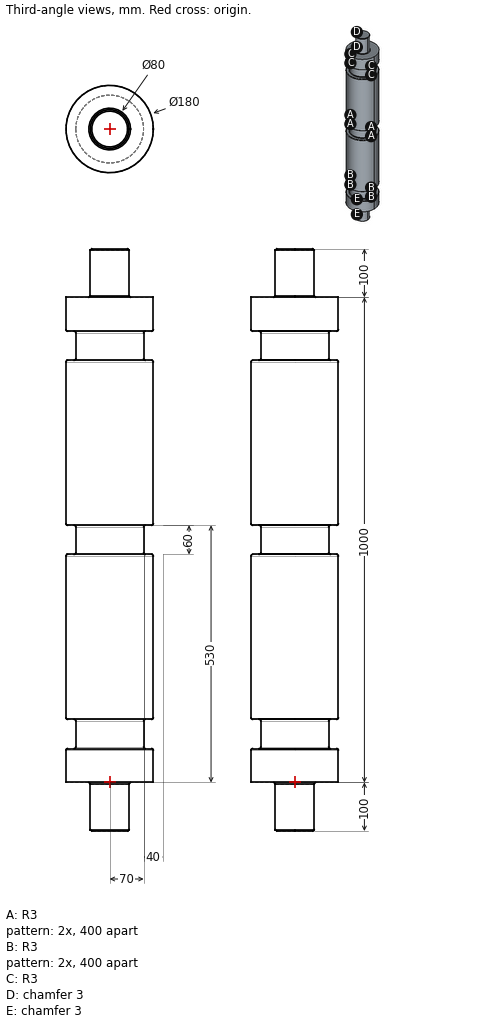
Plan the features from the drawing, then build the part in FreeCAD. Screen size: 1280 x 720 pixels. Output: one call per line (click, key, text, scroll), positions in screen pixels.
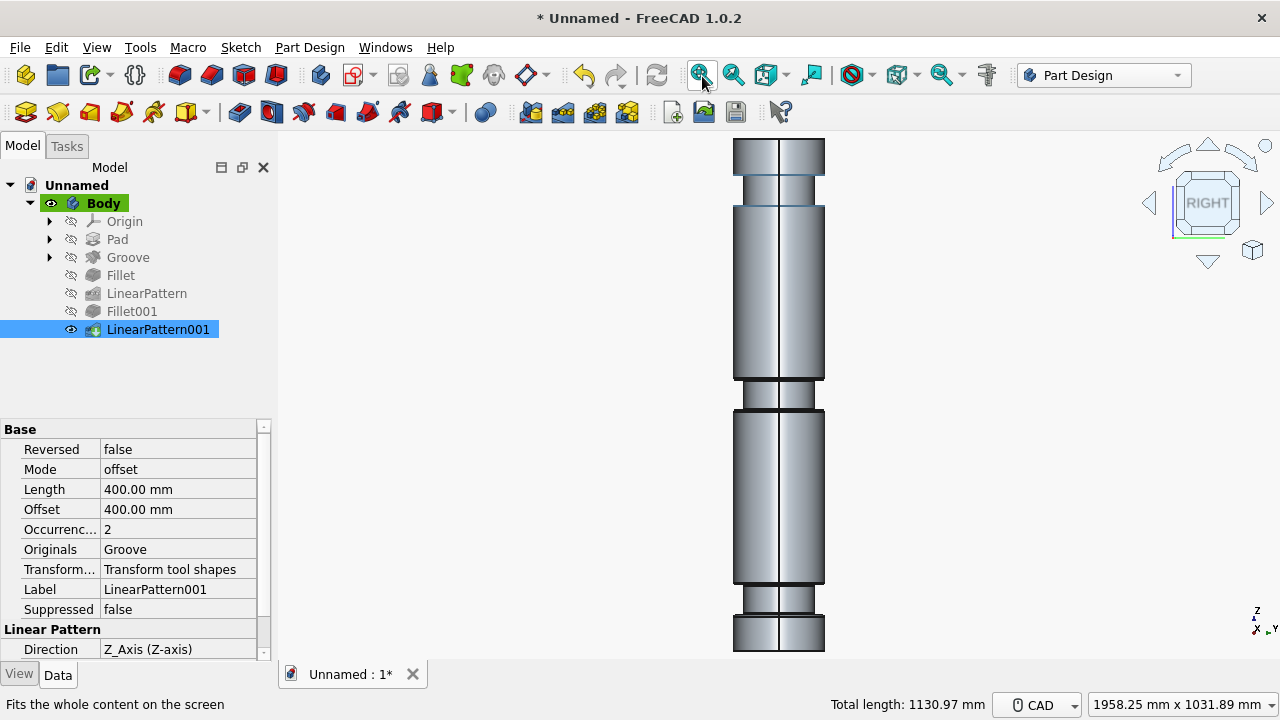
key(5)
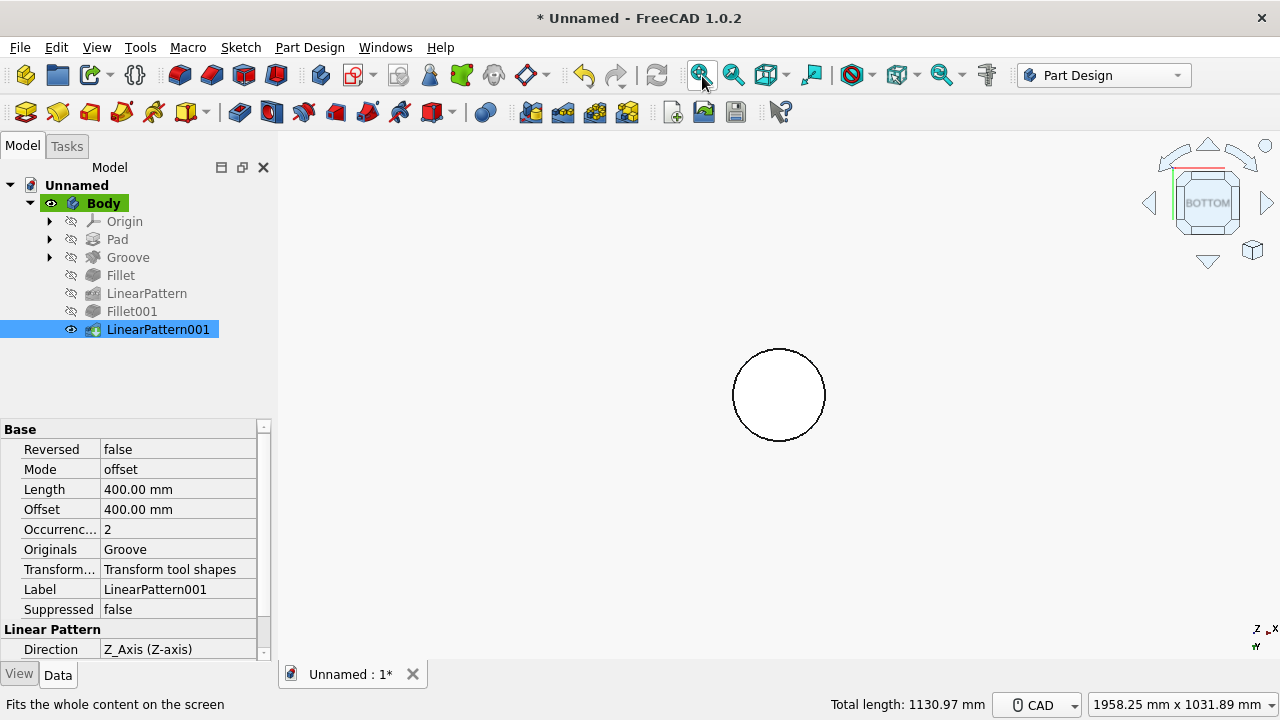
click(702, 76)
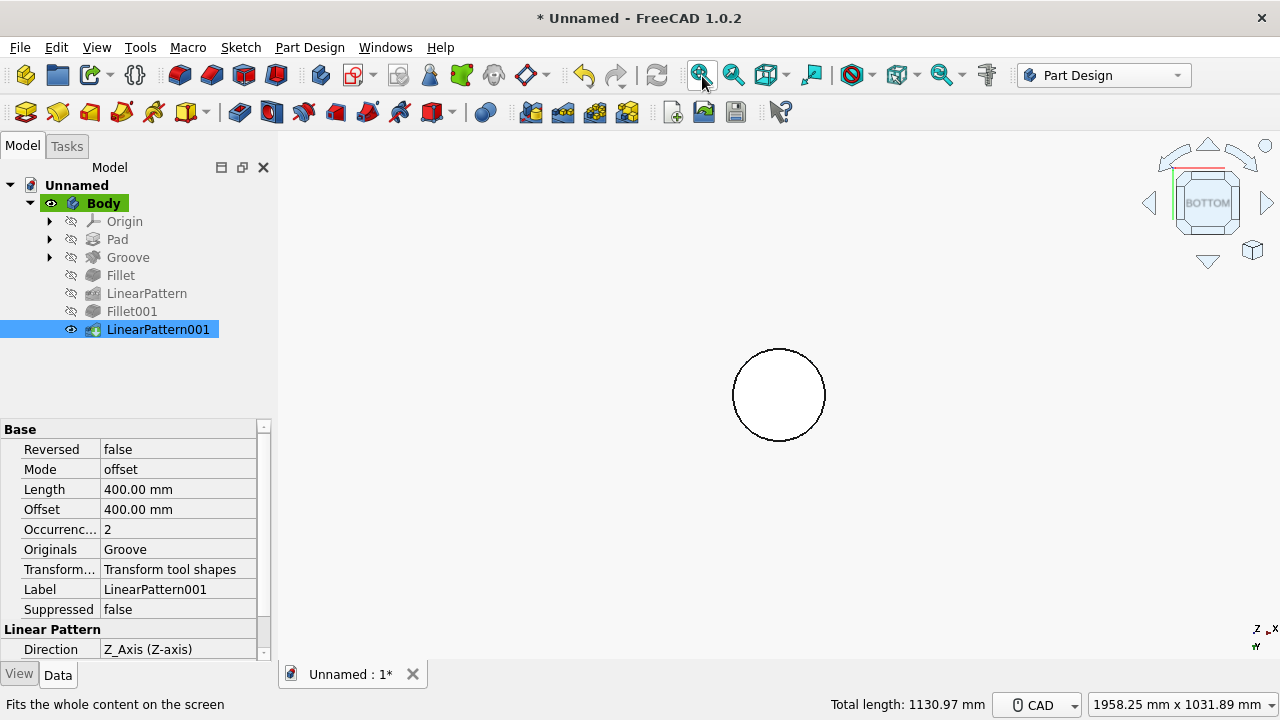
key(4)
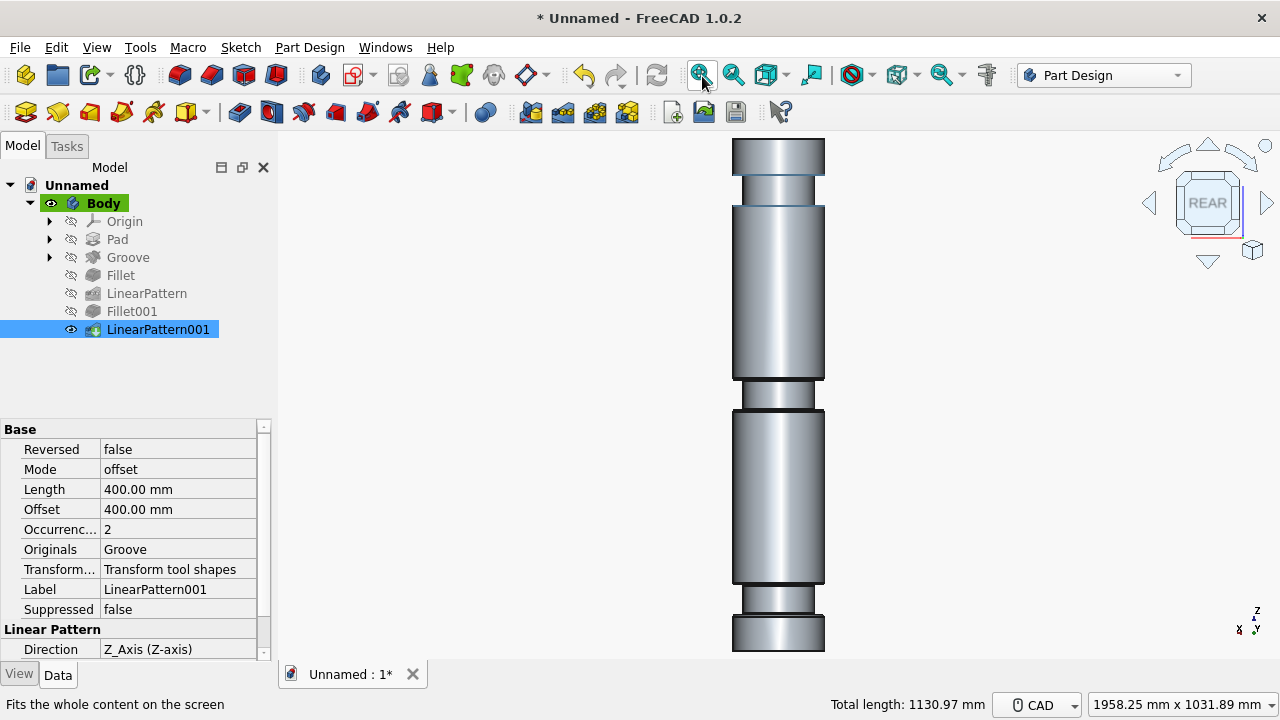
key(6)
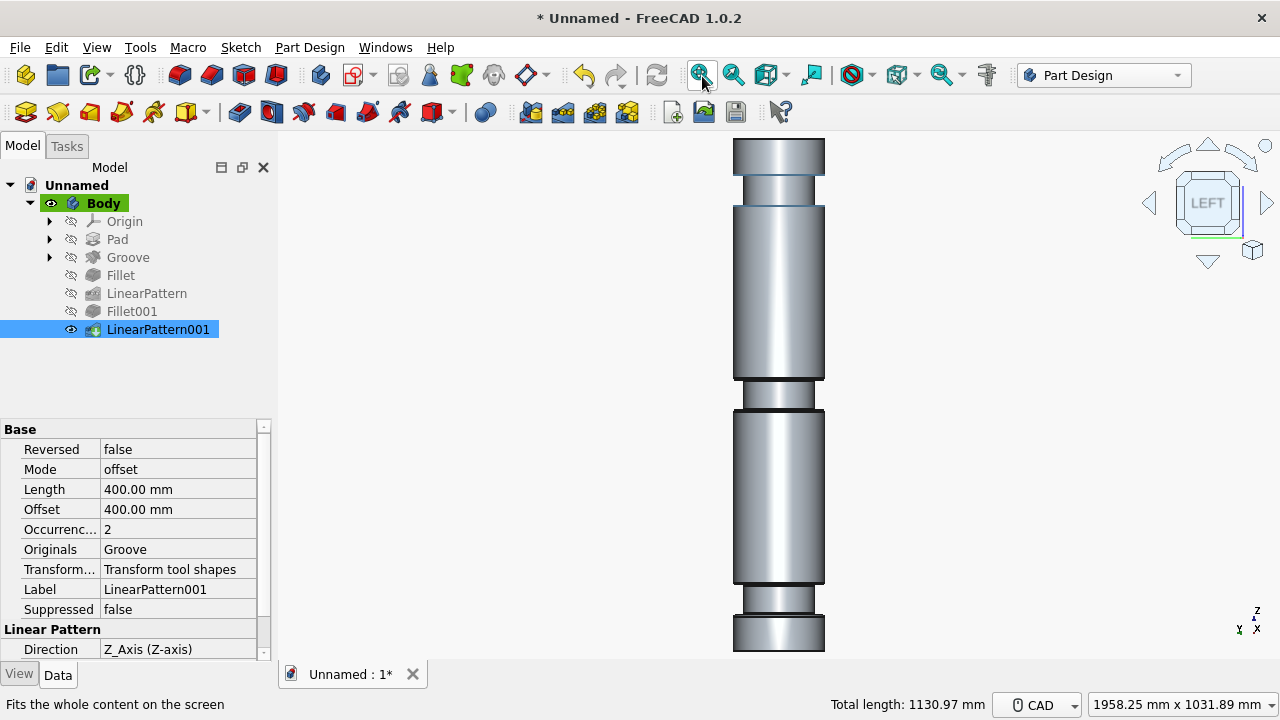
key(v)
key(3)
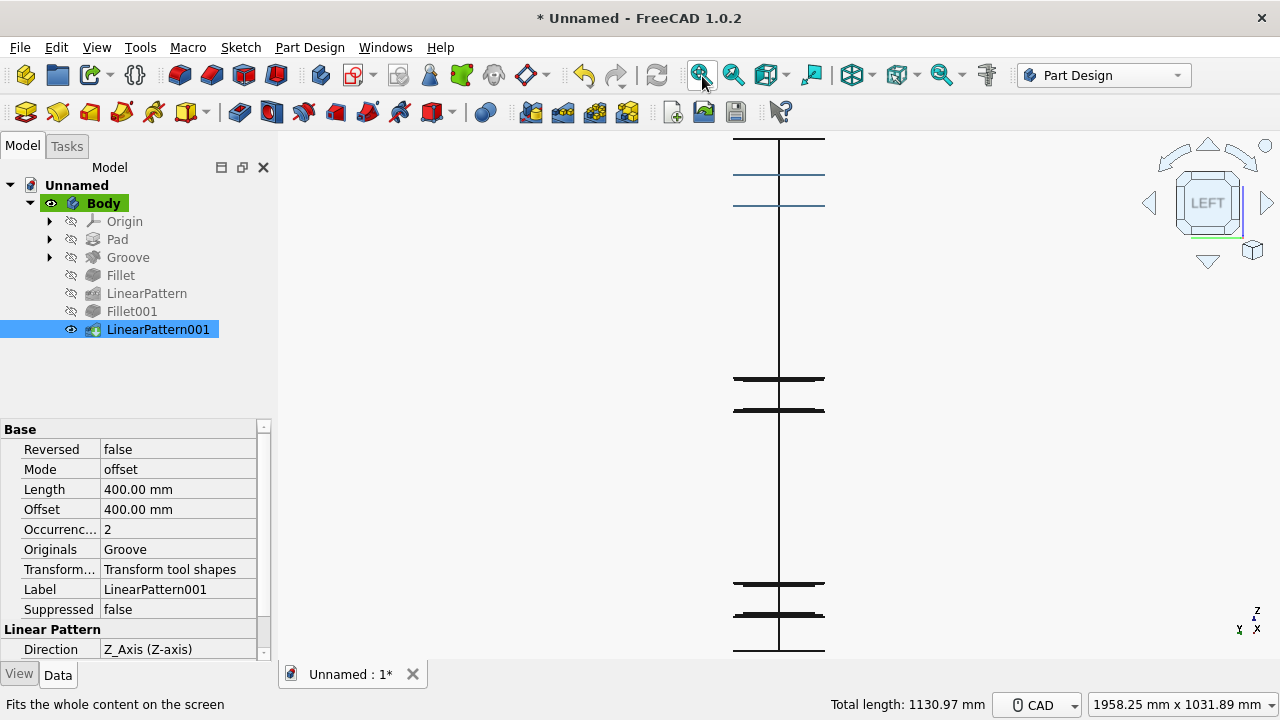
key(0)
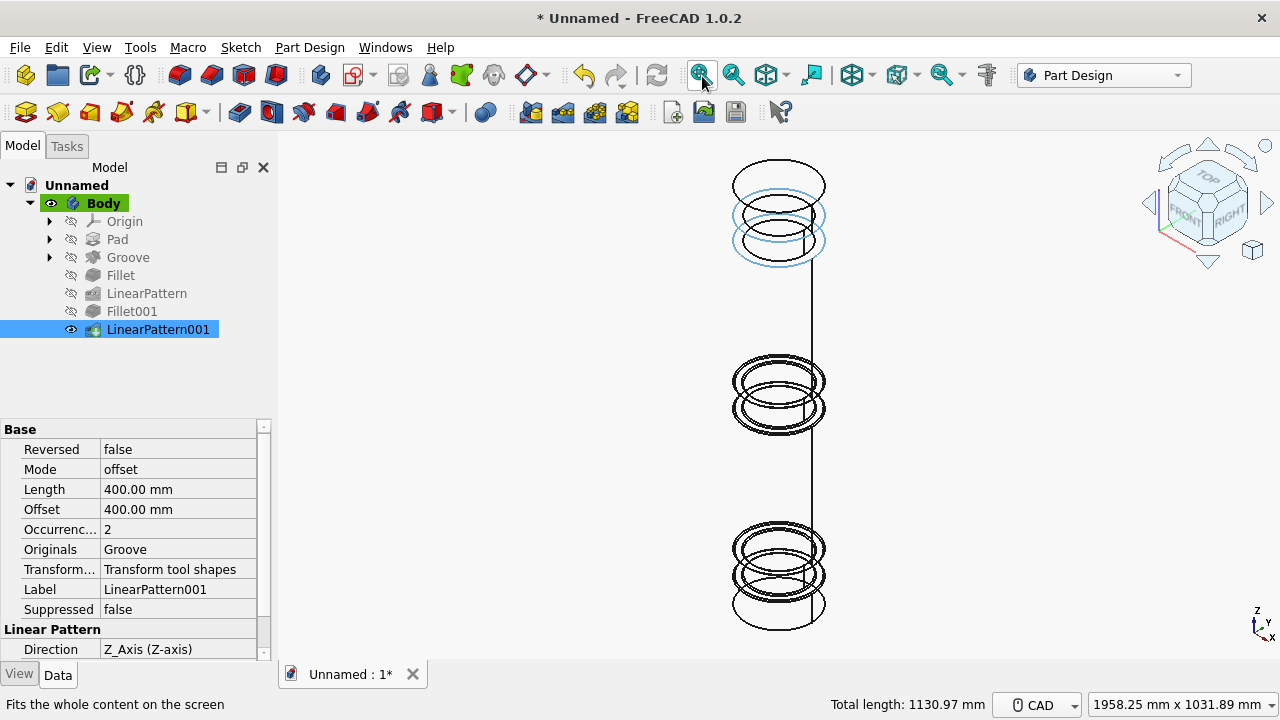
click(754, 200, ctrl)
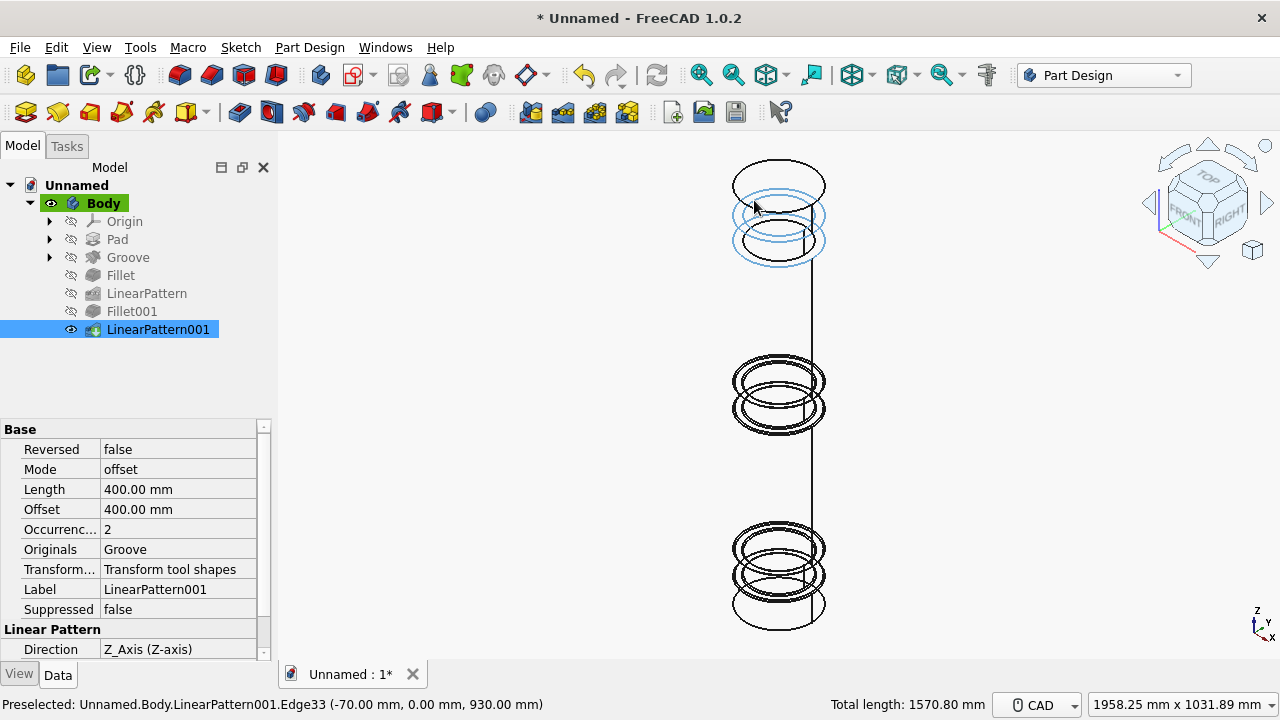
click(773, 219, ctrl)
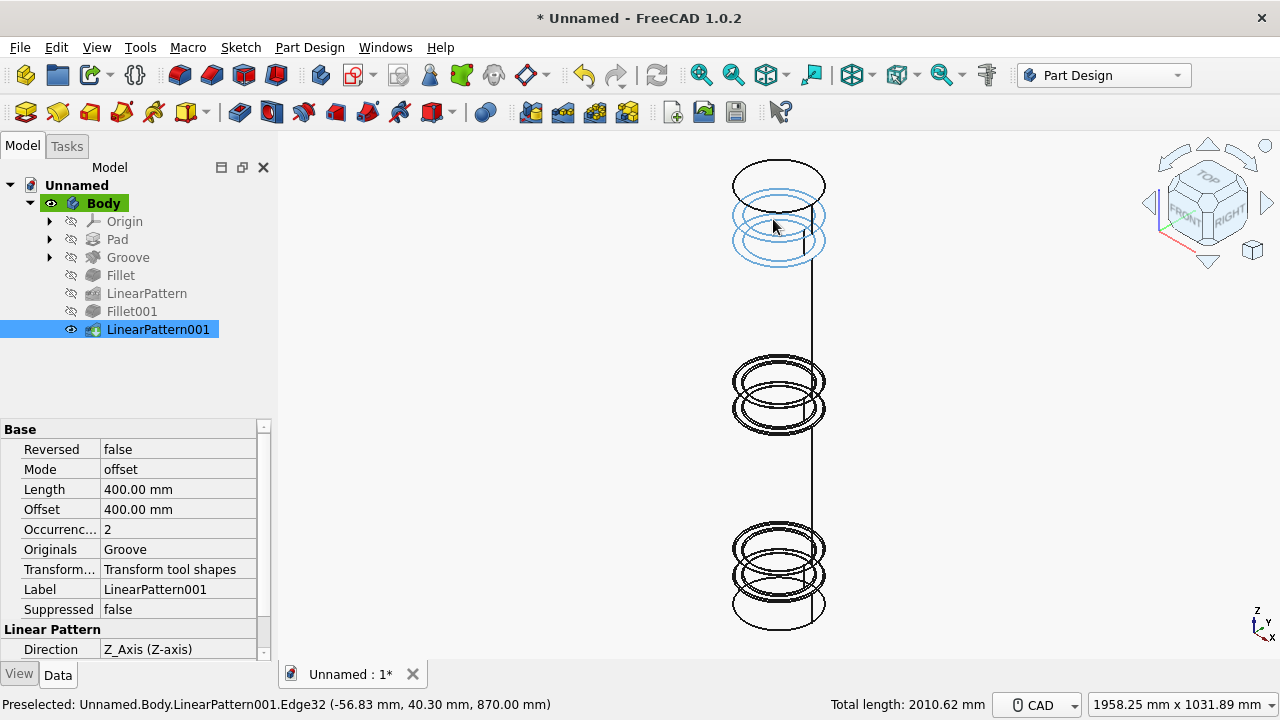
key(v)
key(1)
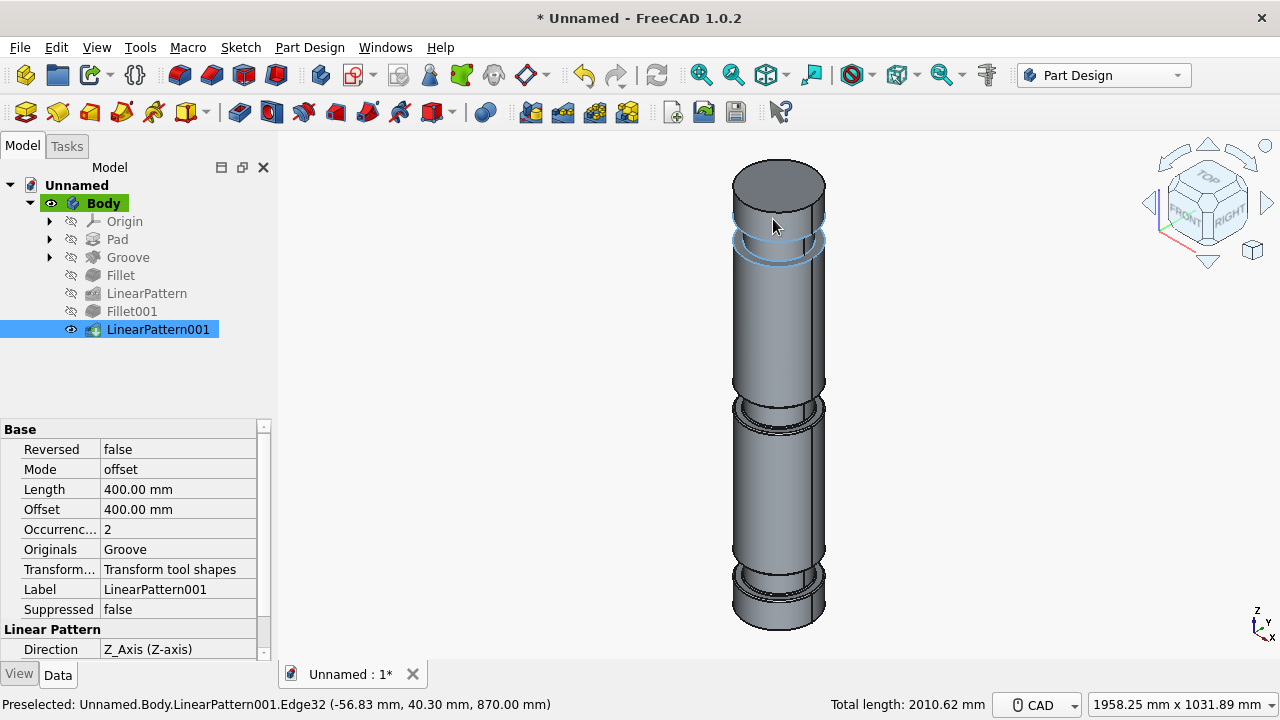
click(180, 76)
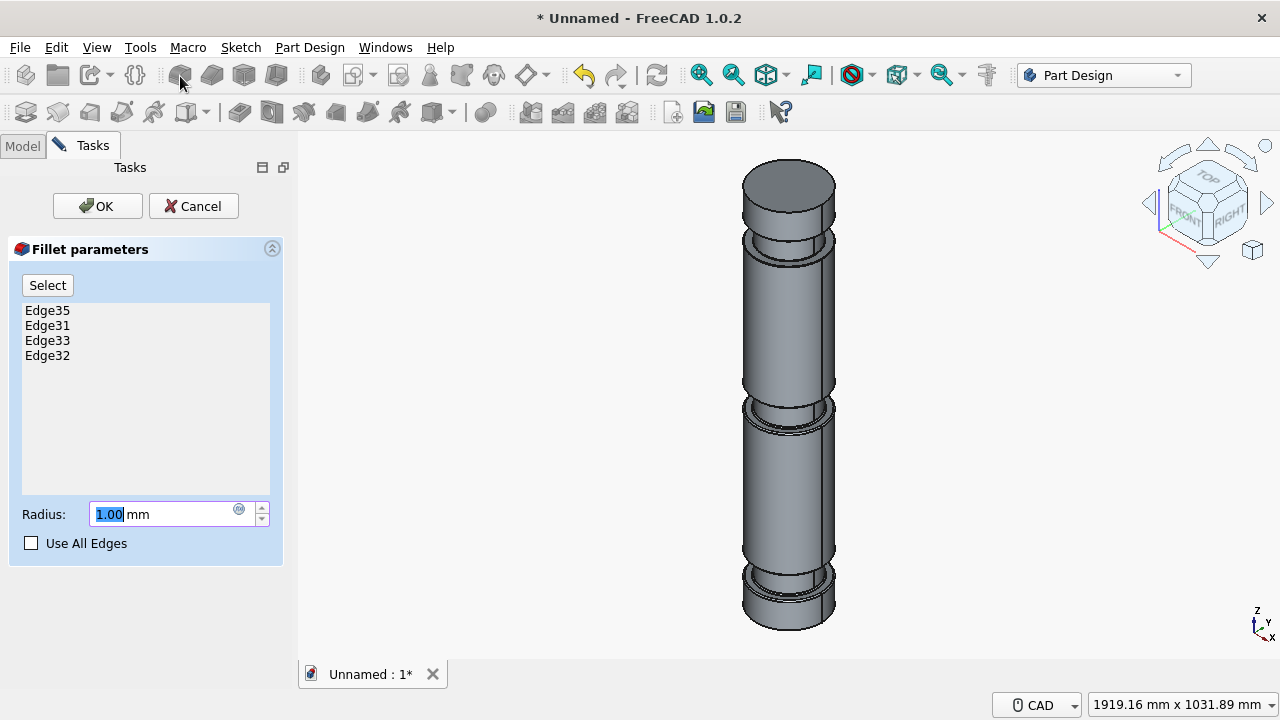
text(3)
key(Tab)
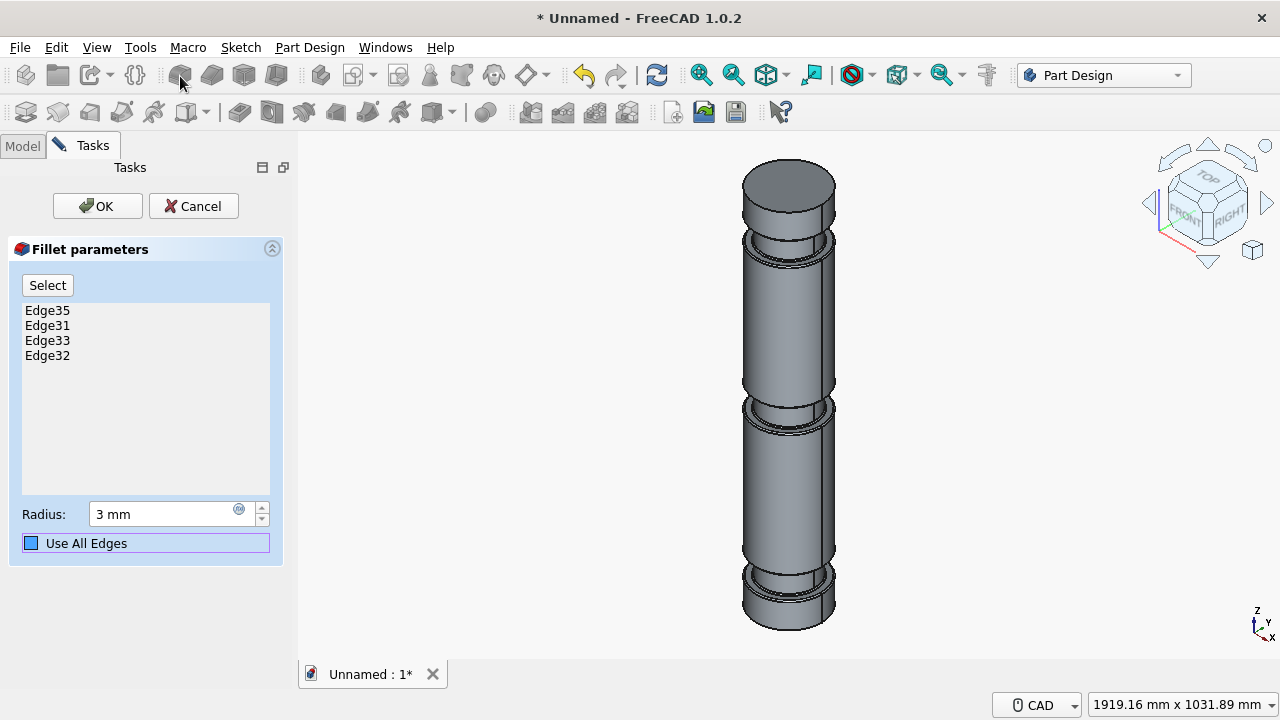
click(98, 206)